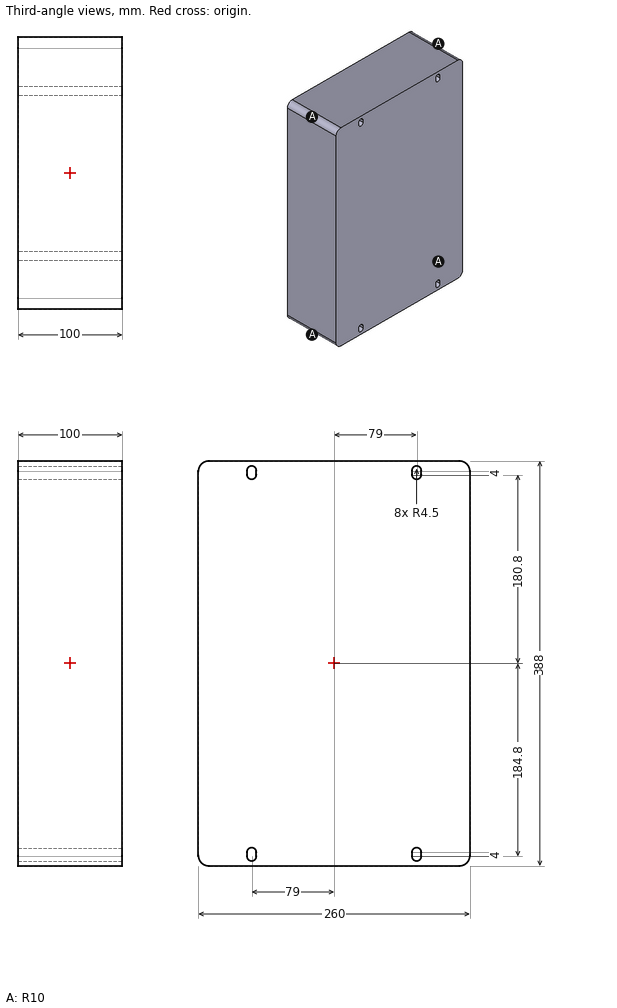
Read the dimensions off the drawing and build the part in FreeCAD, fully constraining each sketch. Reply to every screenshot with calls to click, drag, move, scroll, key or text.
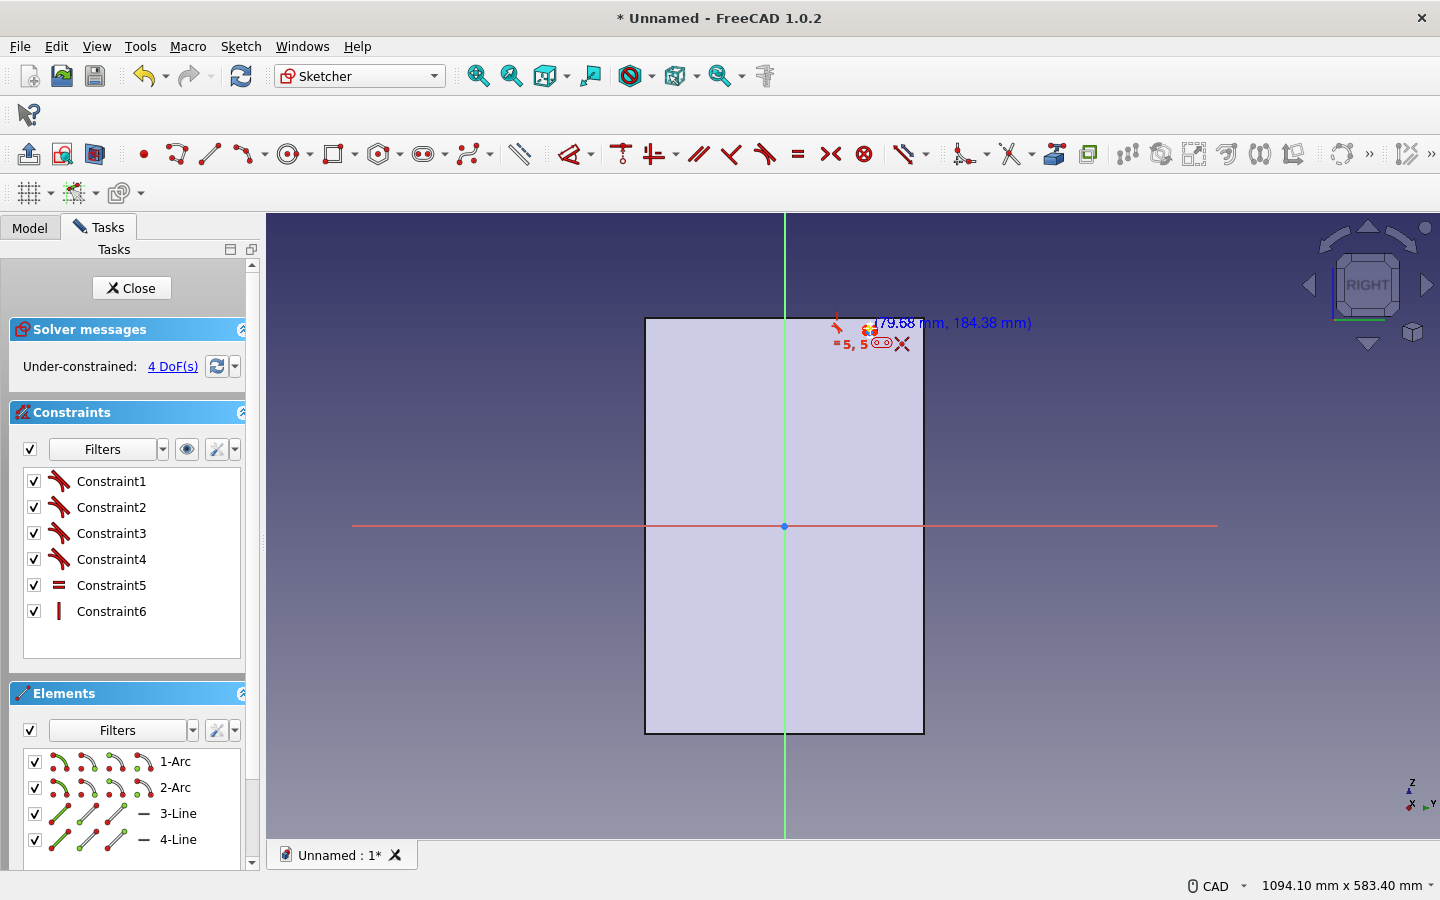
scroll(870, 725, up, 8)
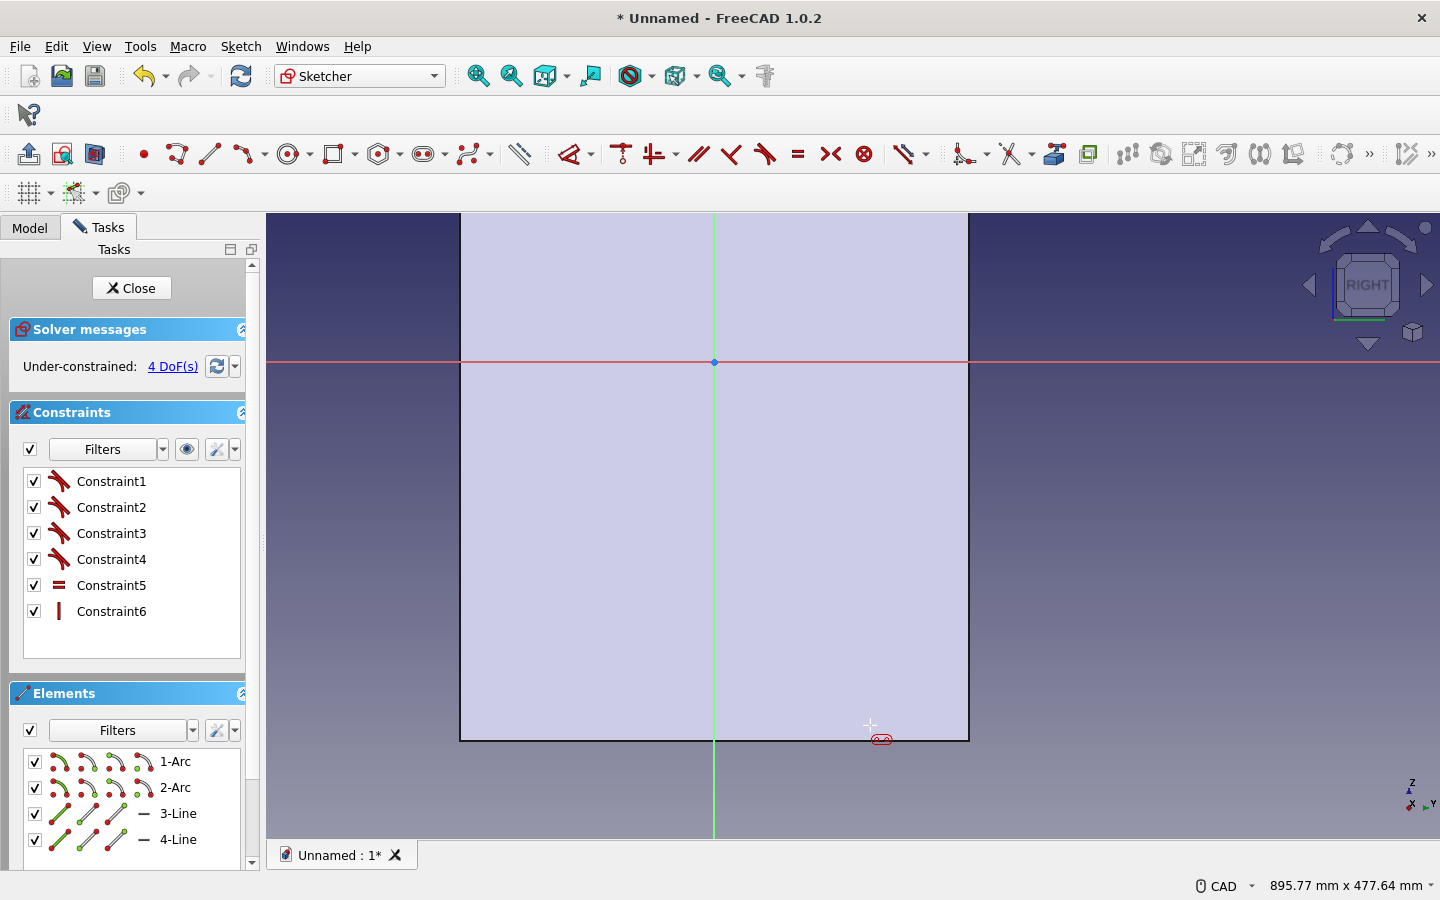
scroll(870, 726, down, 8)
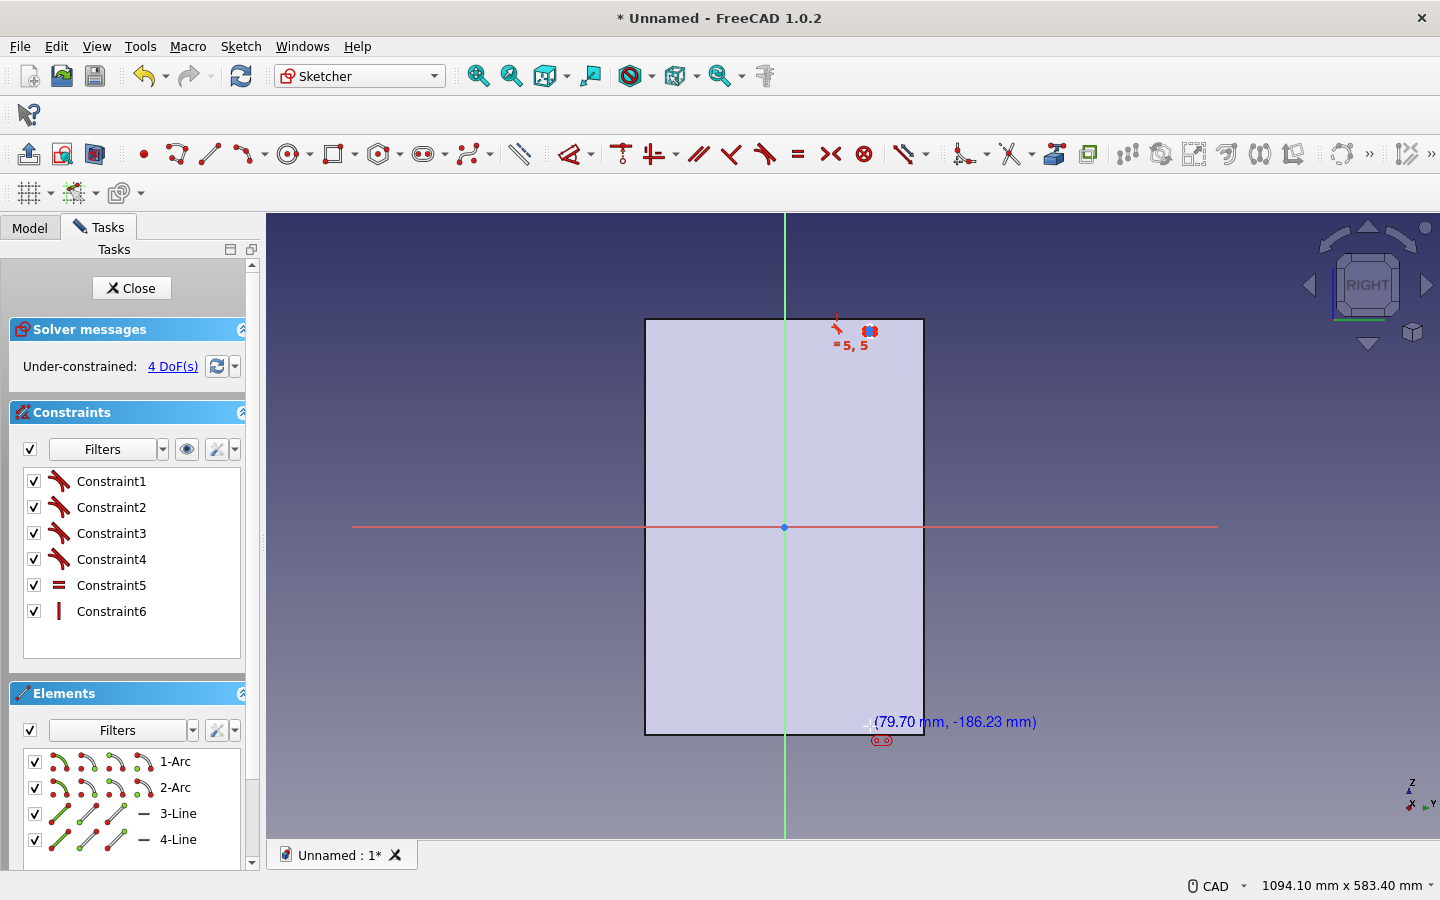
click(870, 725)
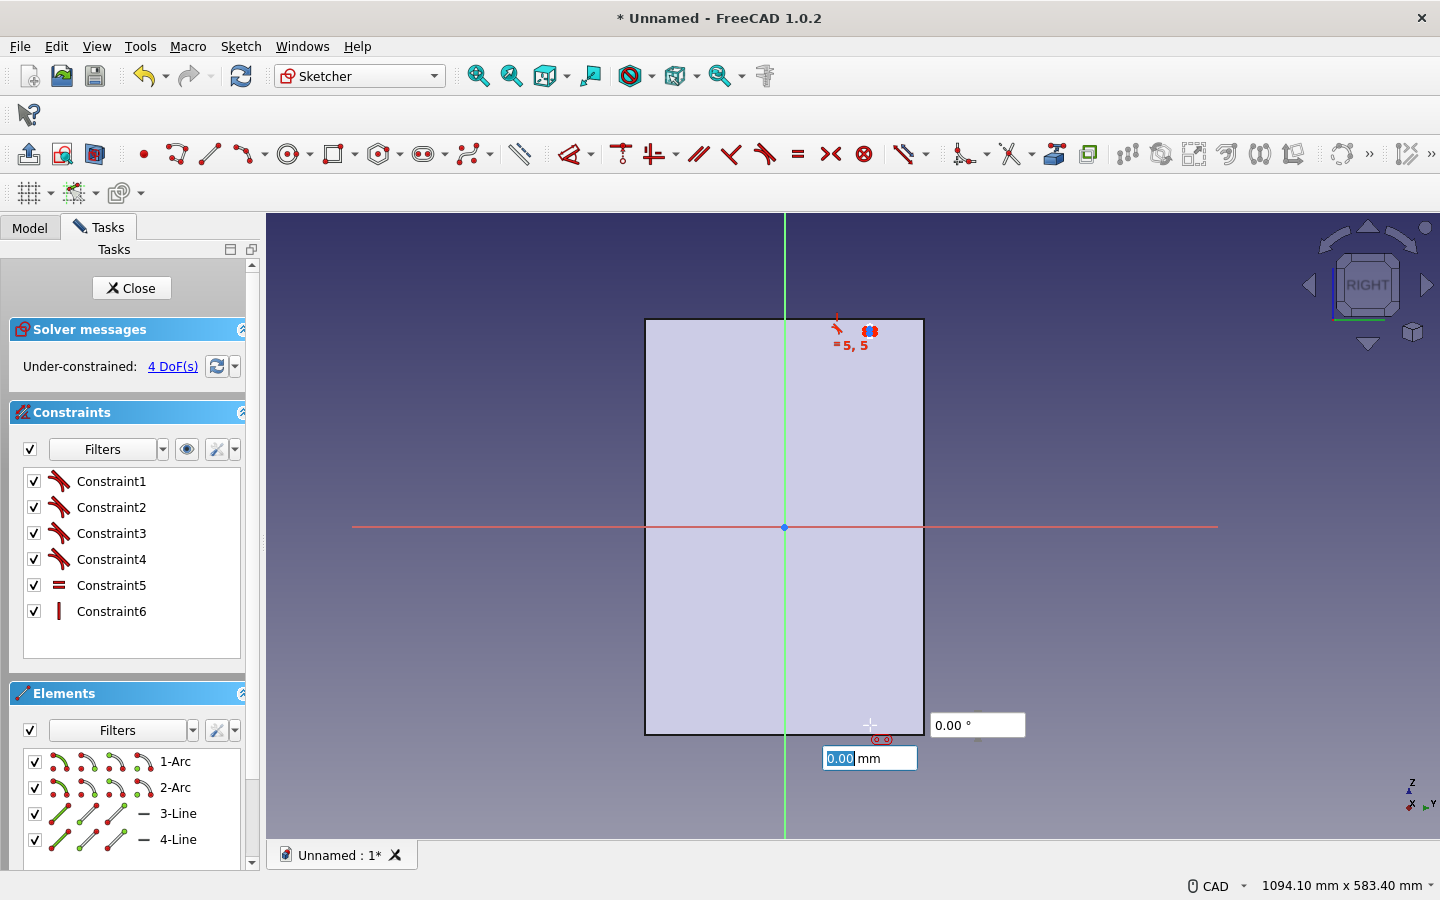
scroll(870, 721, up, 7)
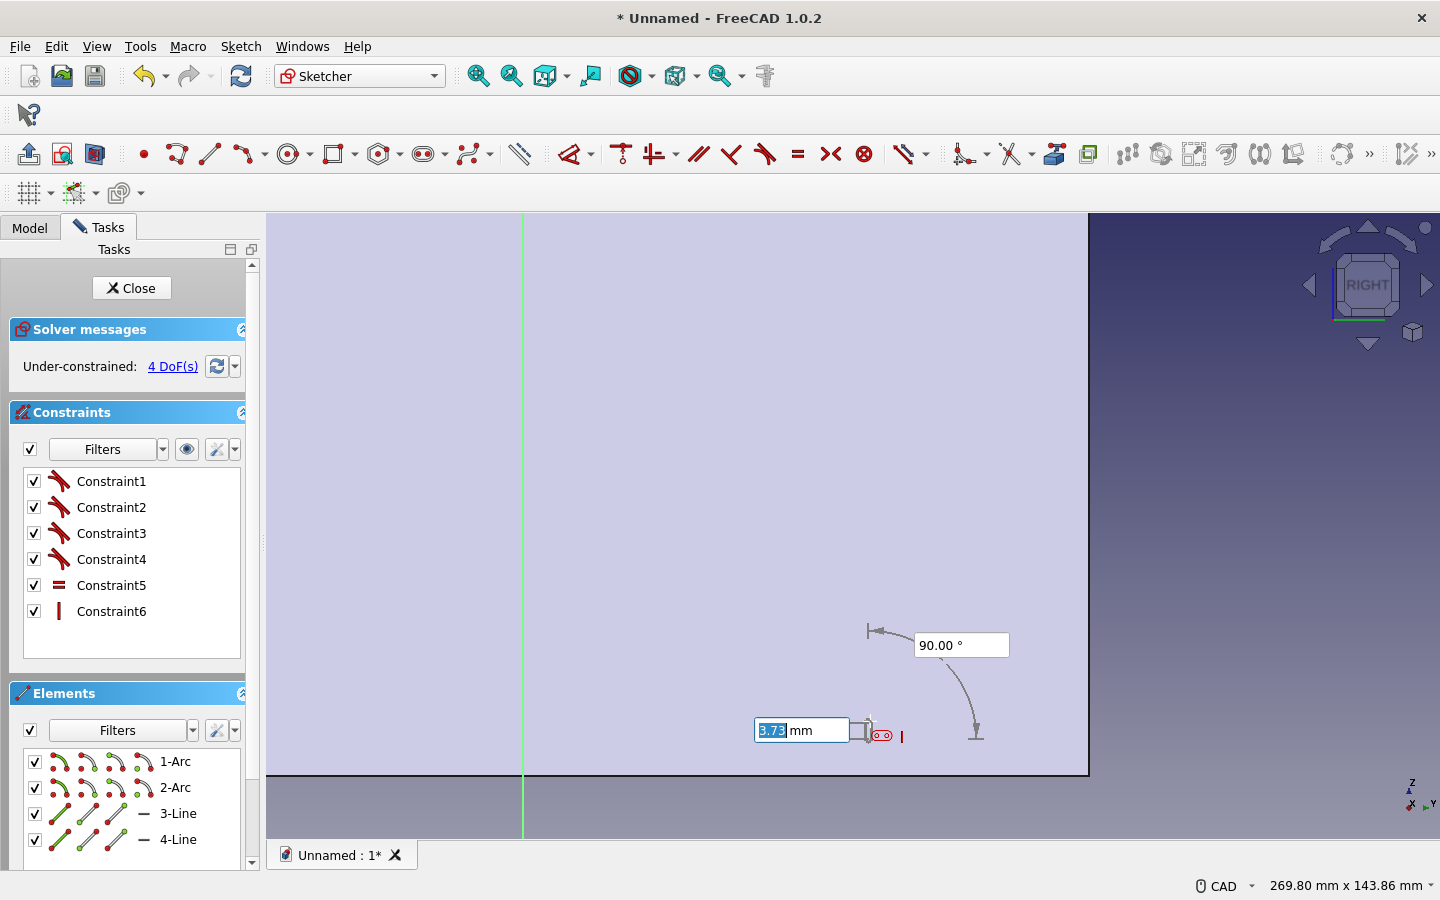
click(868, 719)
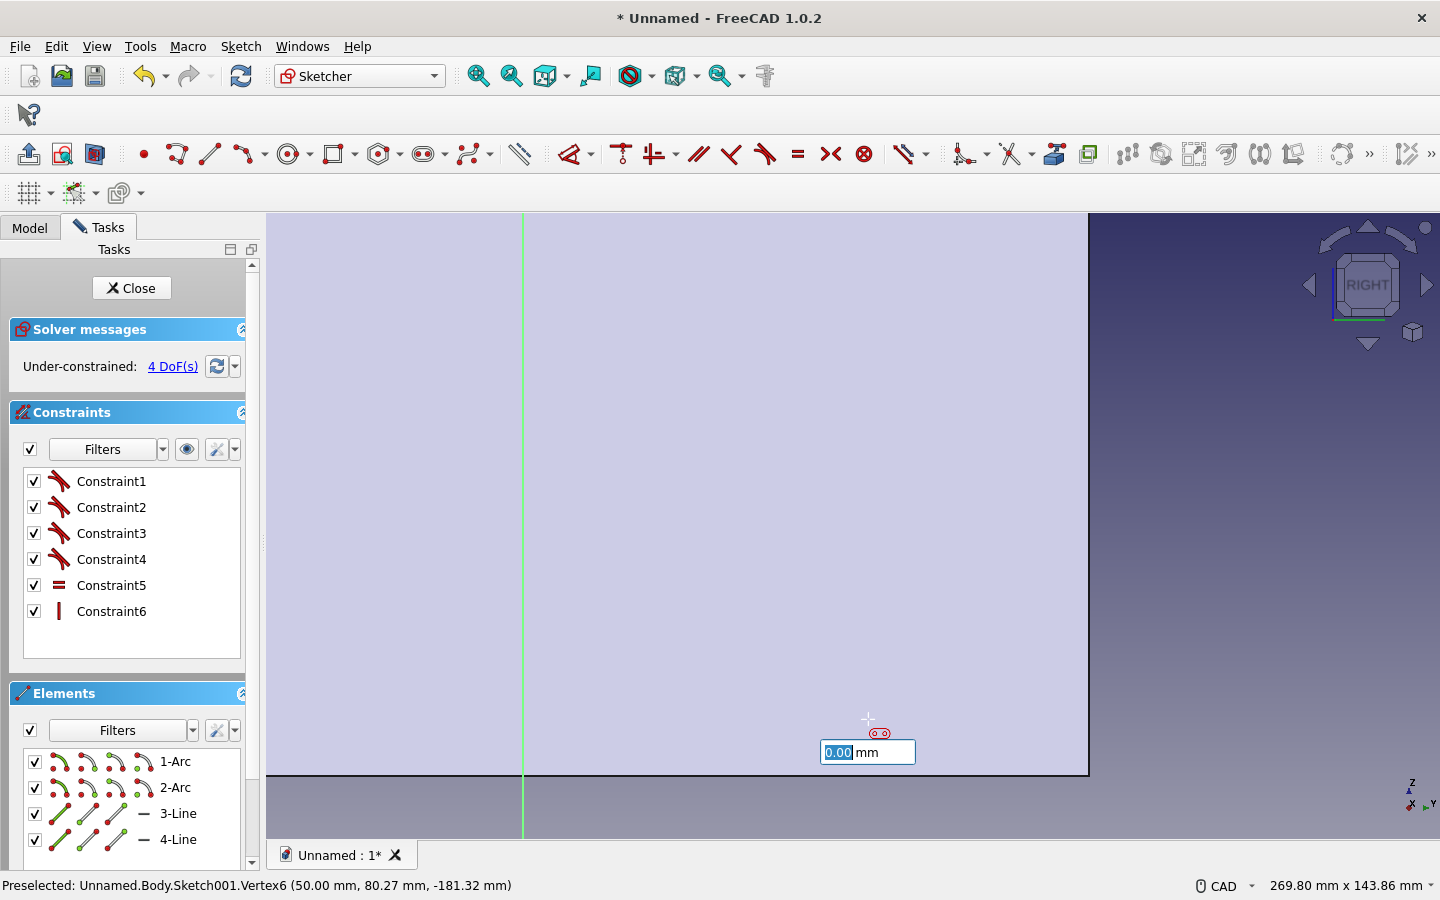
click(887, 727)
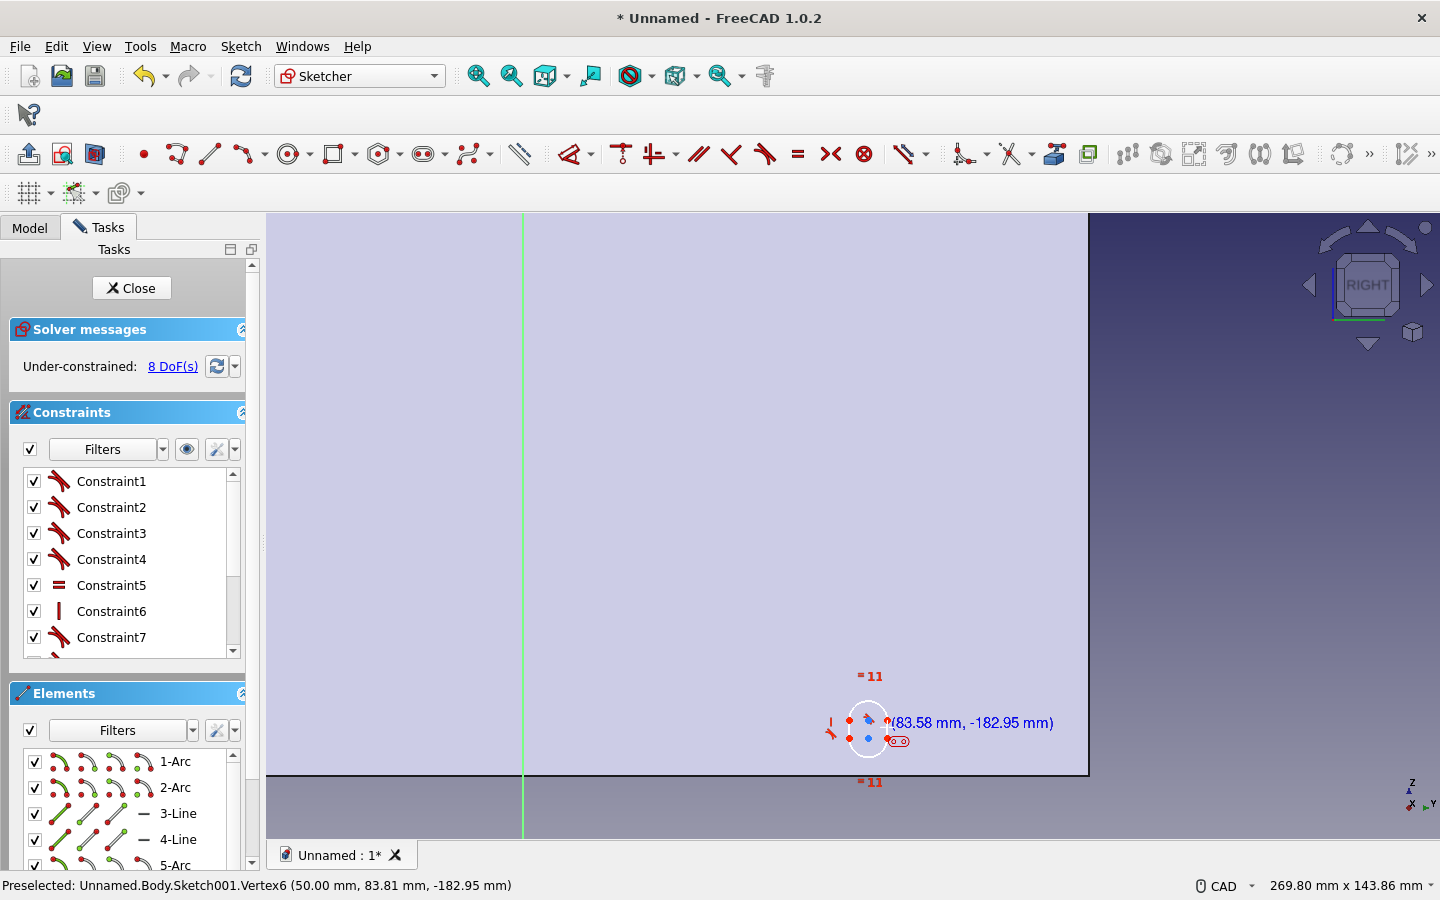
scroll(870, 720, down, 7)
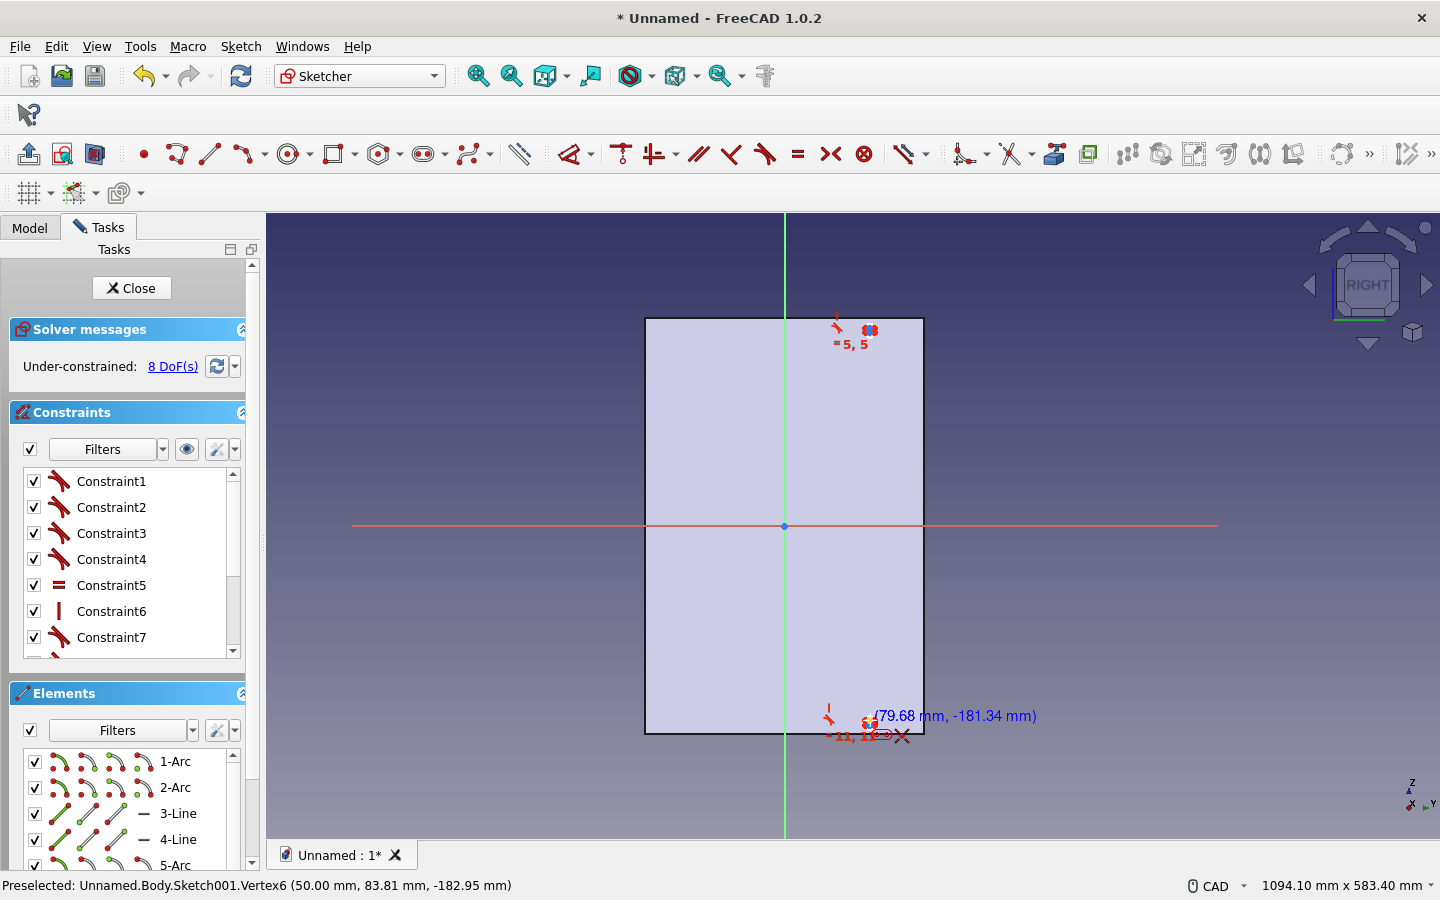
scroll(700, 725, up, 8)